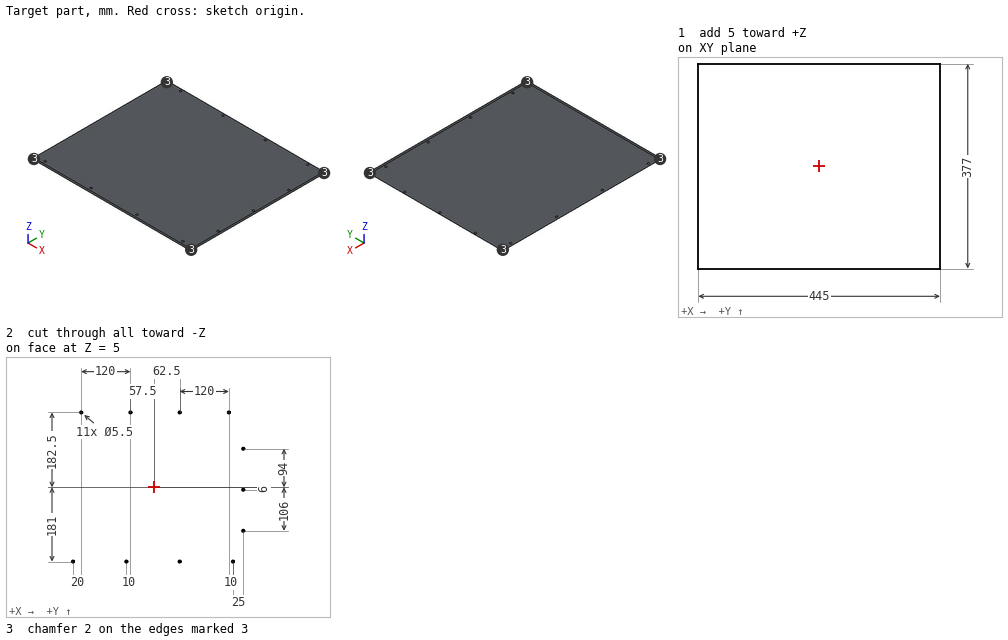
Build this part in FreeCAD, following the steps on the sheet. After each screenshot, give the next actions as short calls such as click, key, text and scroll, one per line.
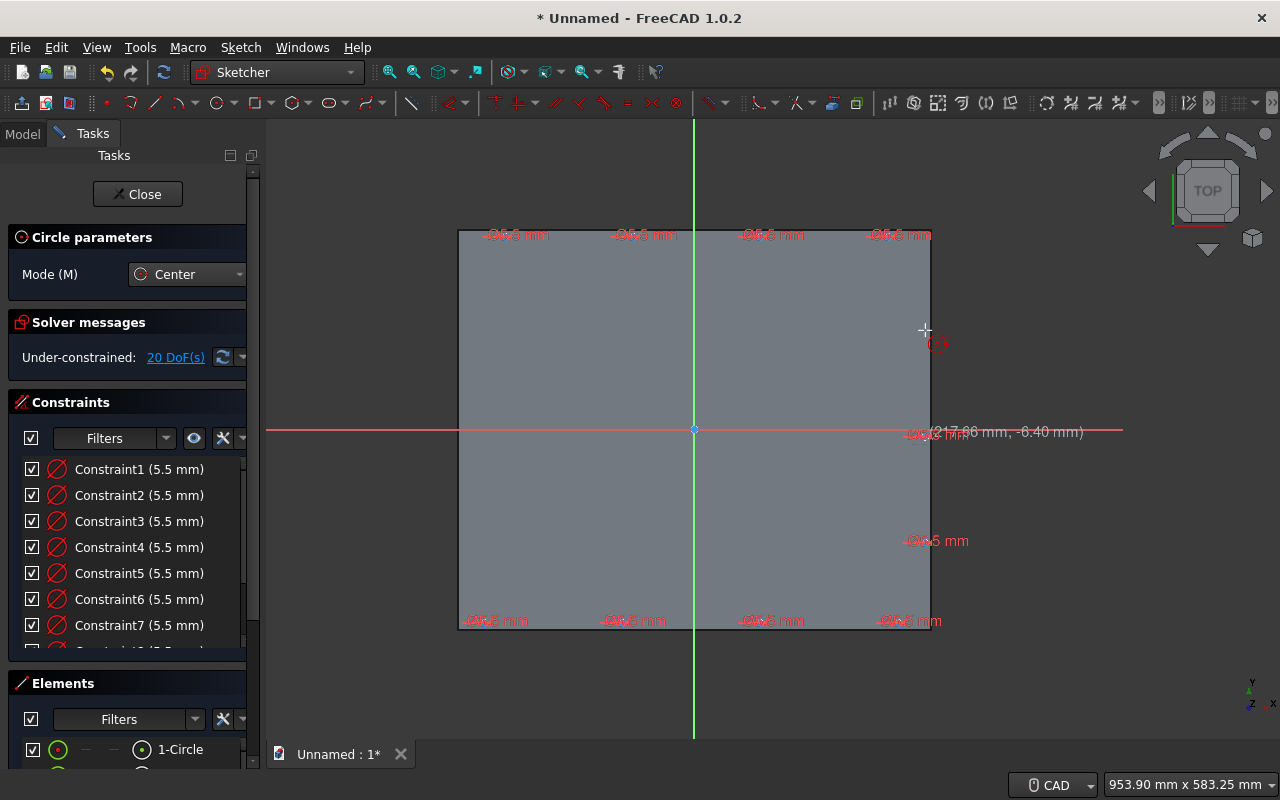
click(925, 330)
move(927, 328)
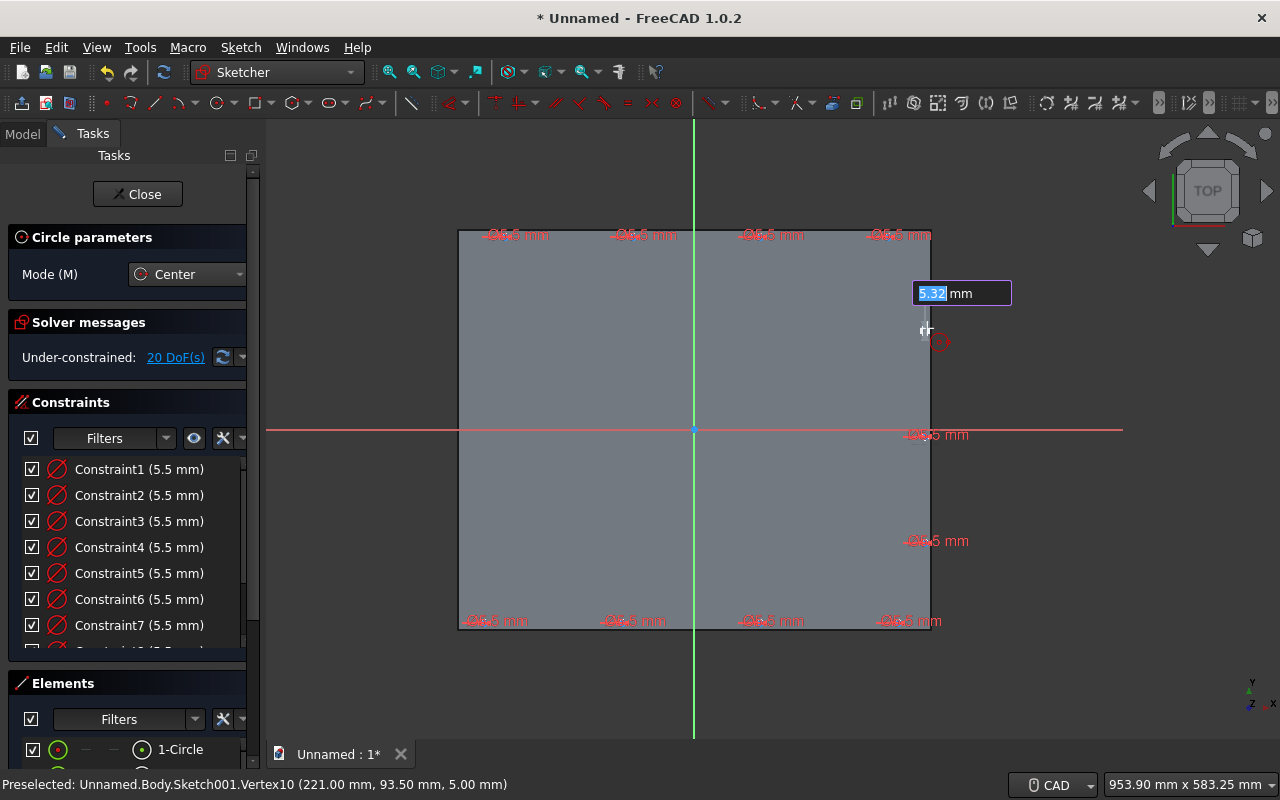
text(5.5)
key(Return)
key(Escape)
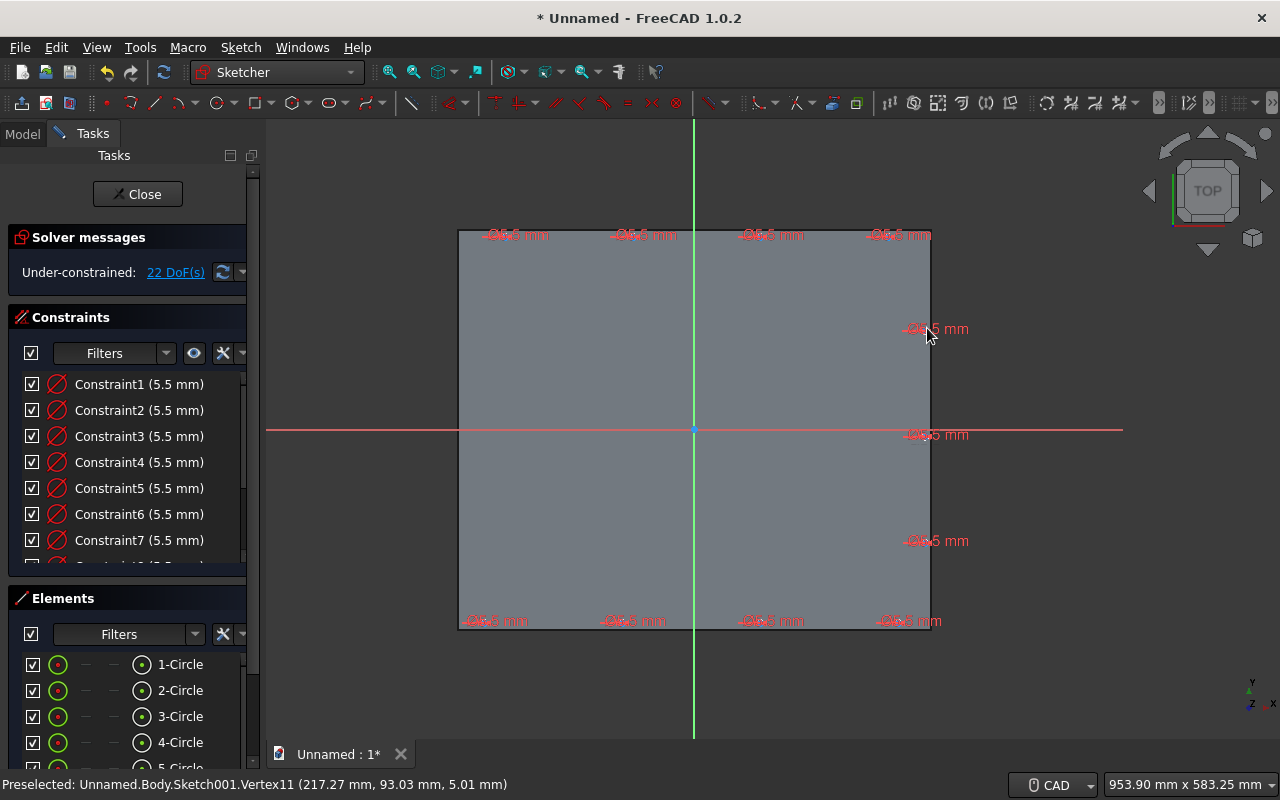
click(505, 237)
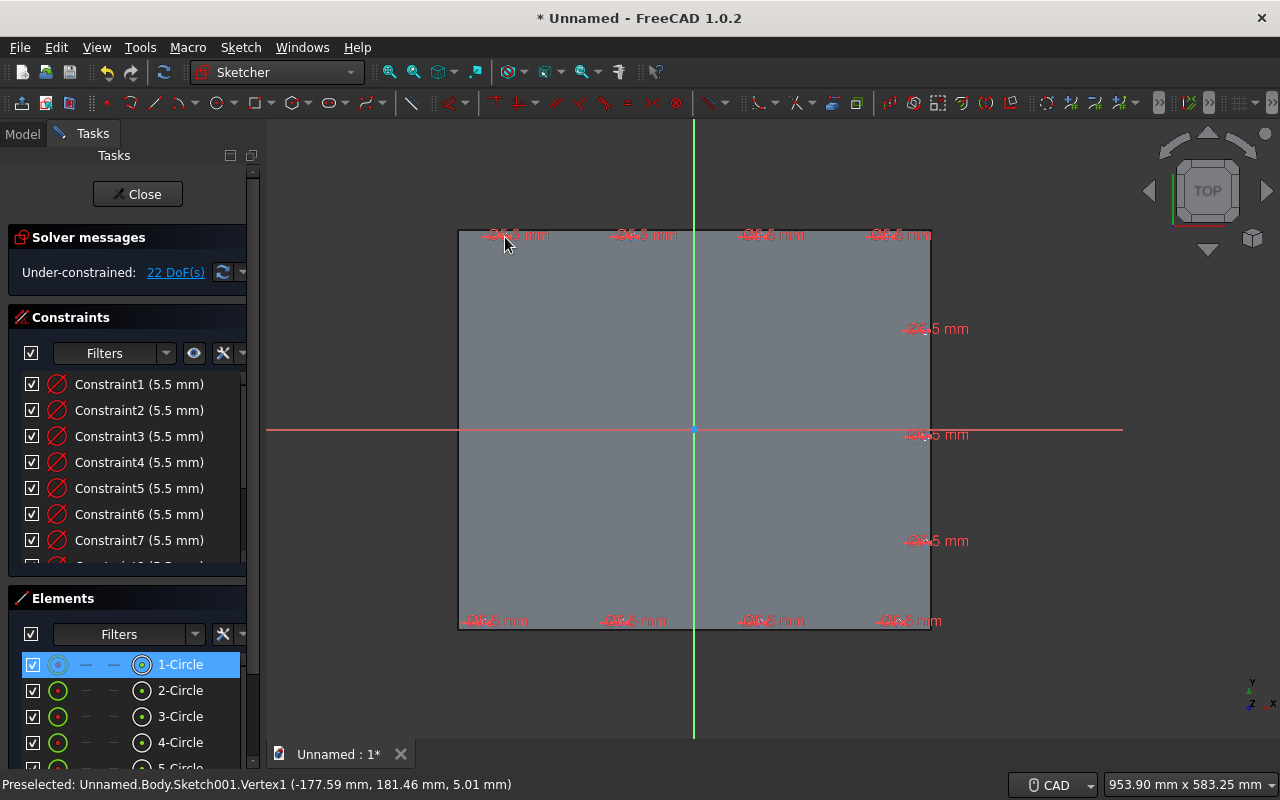
click(633, 237)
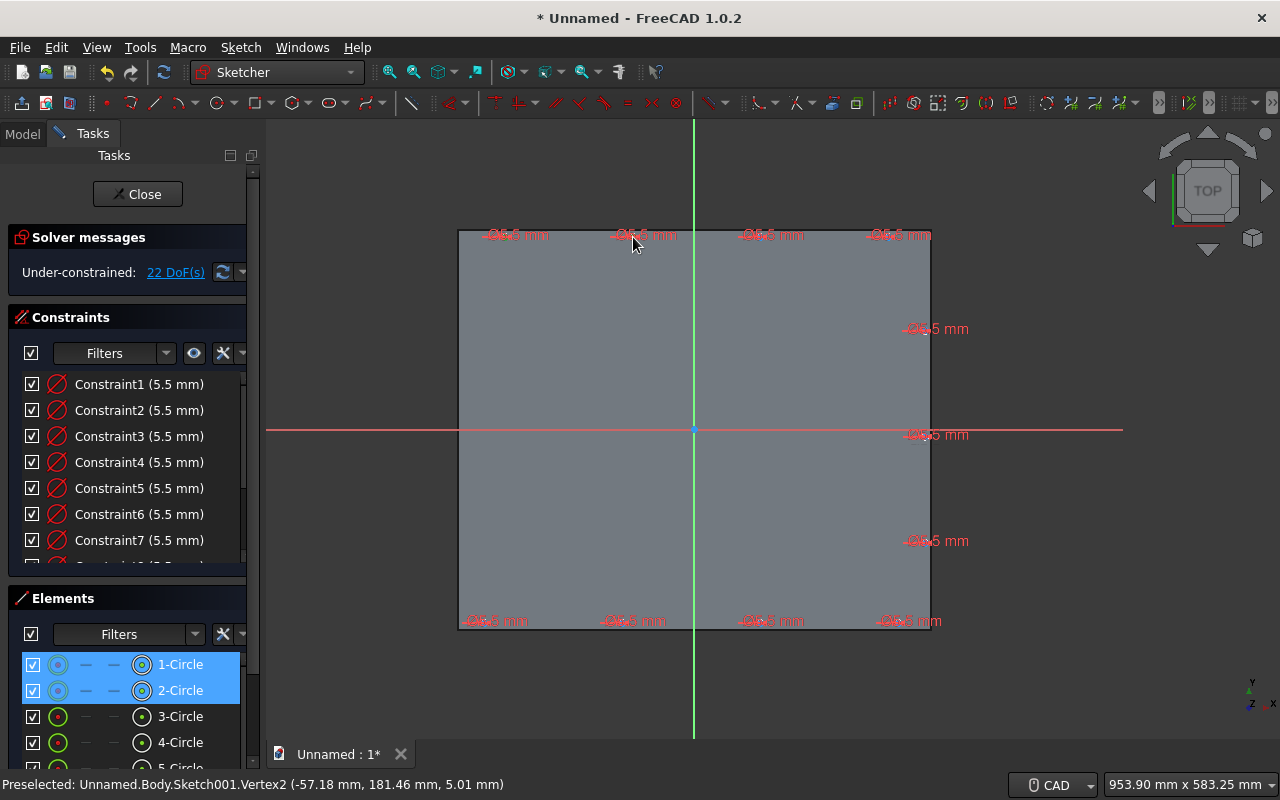
key(h)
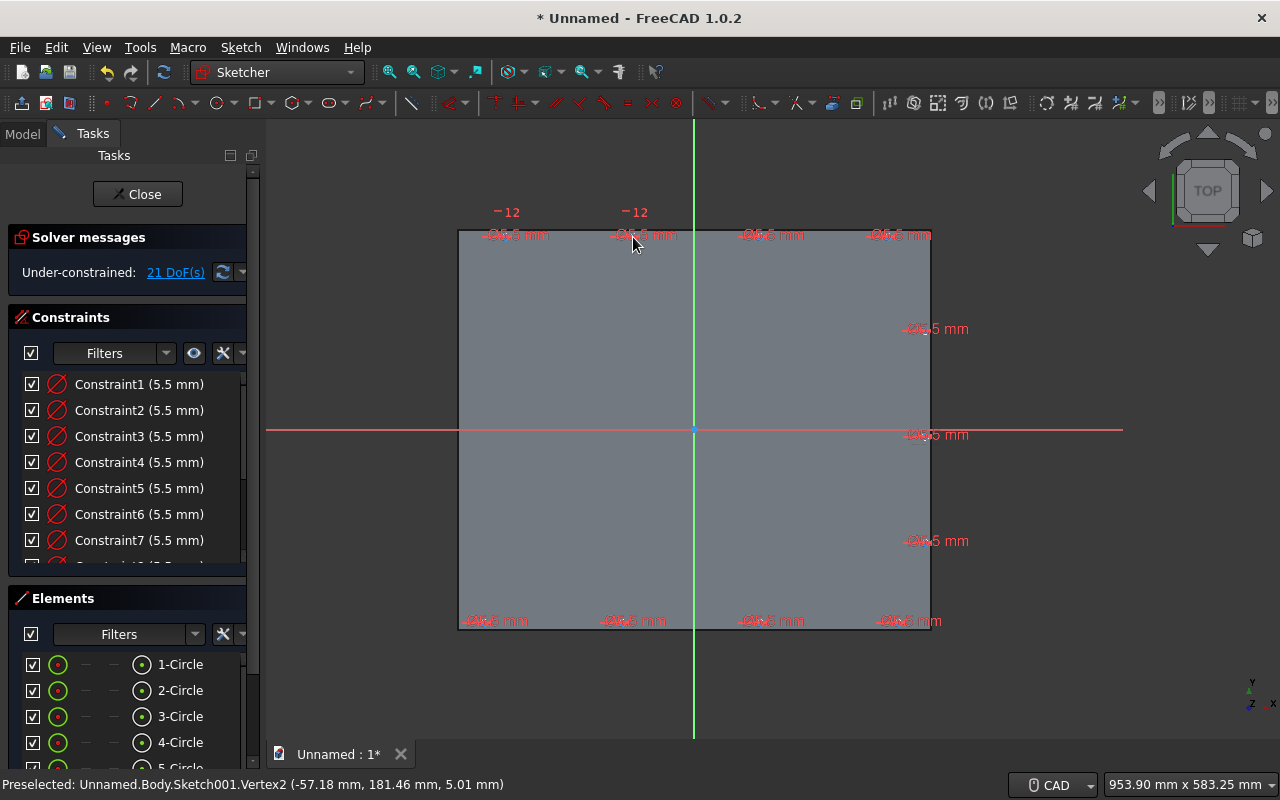
click(633, 237)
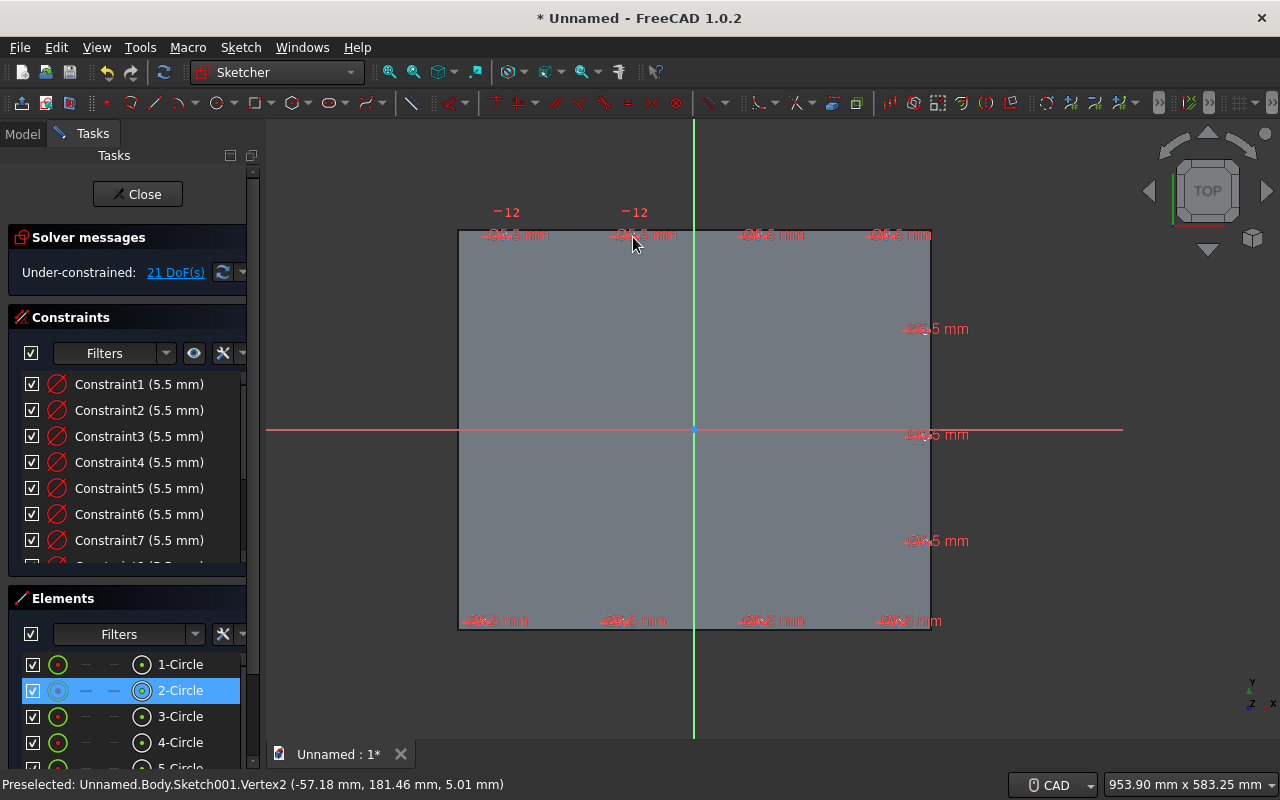
click(760, 237)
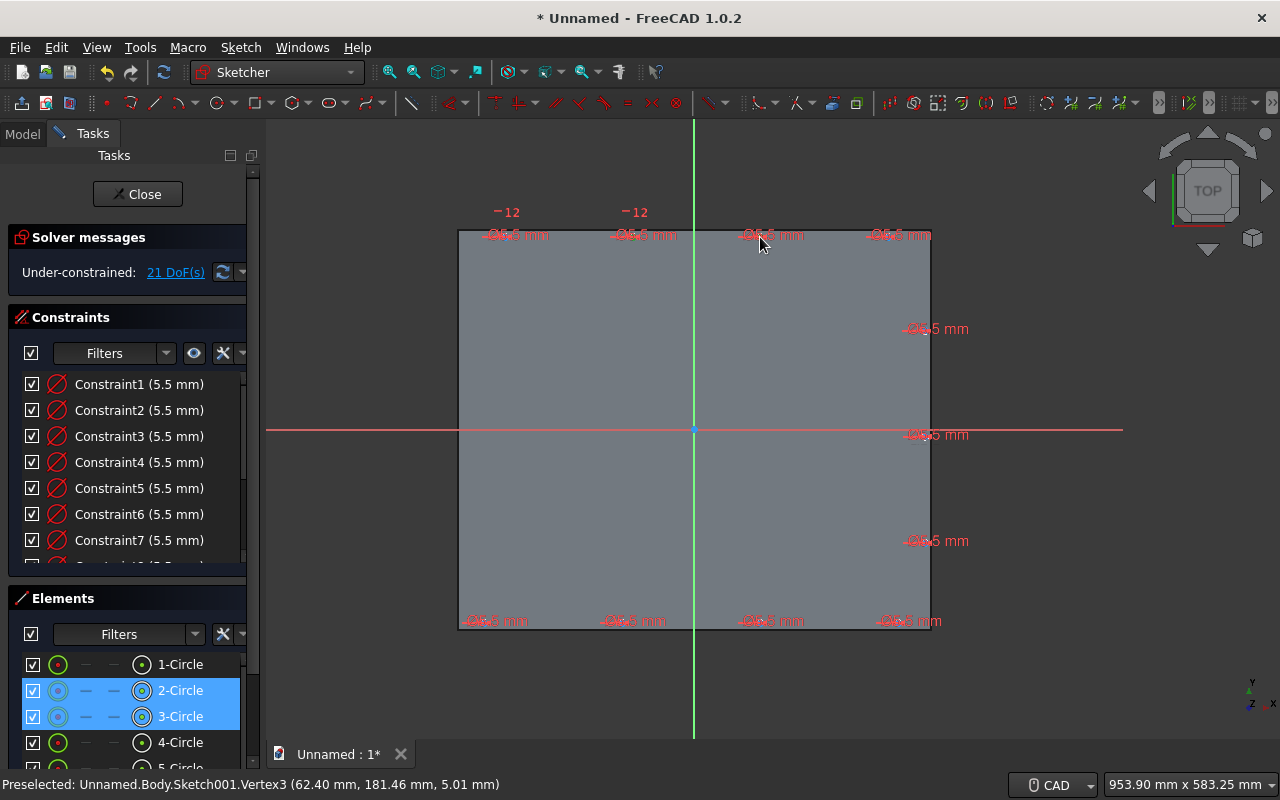
click(538, 104)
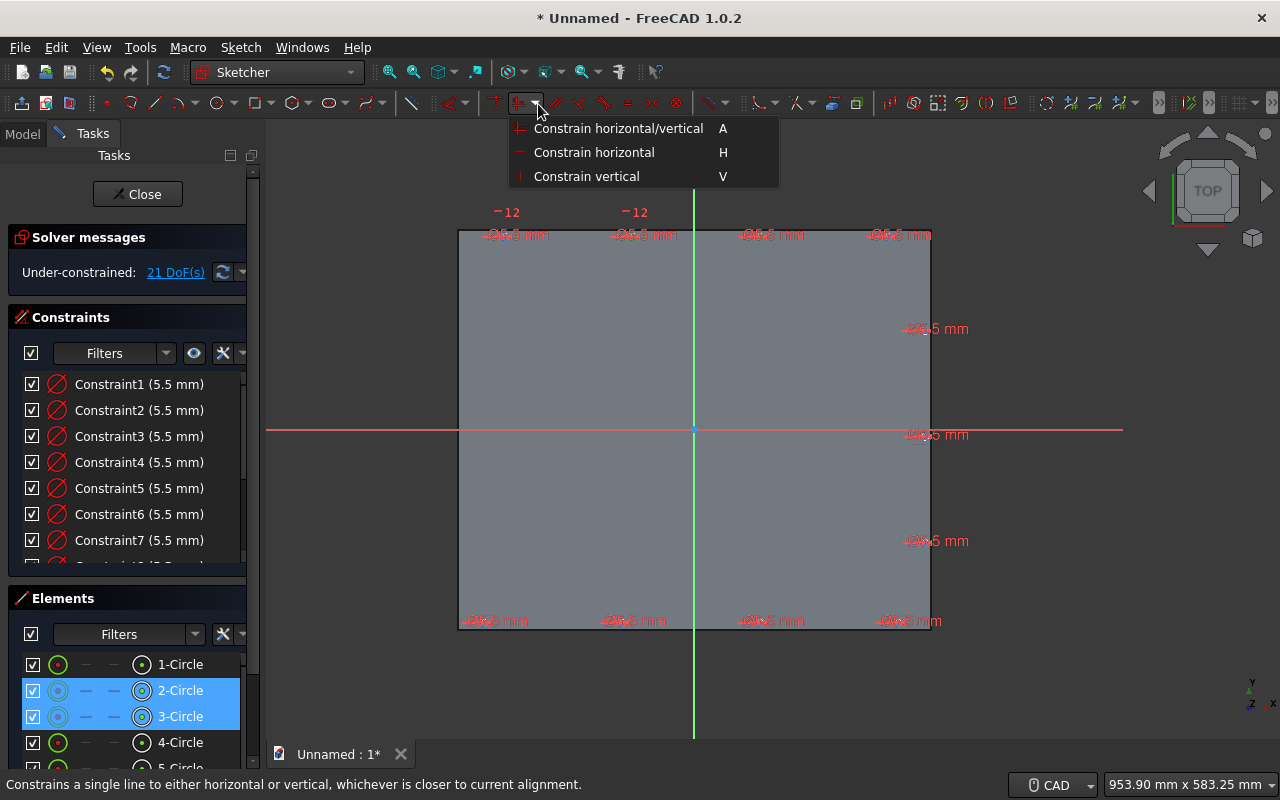
click(644, 152)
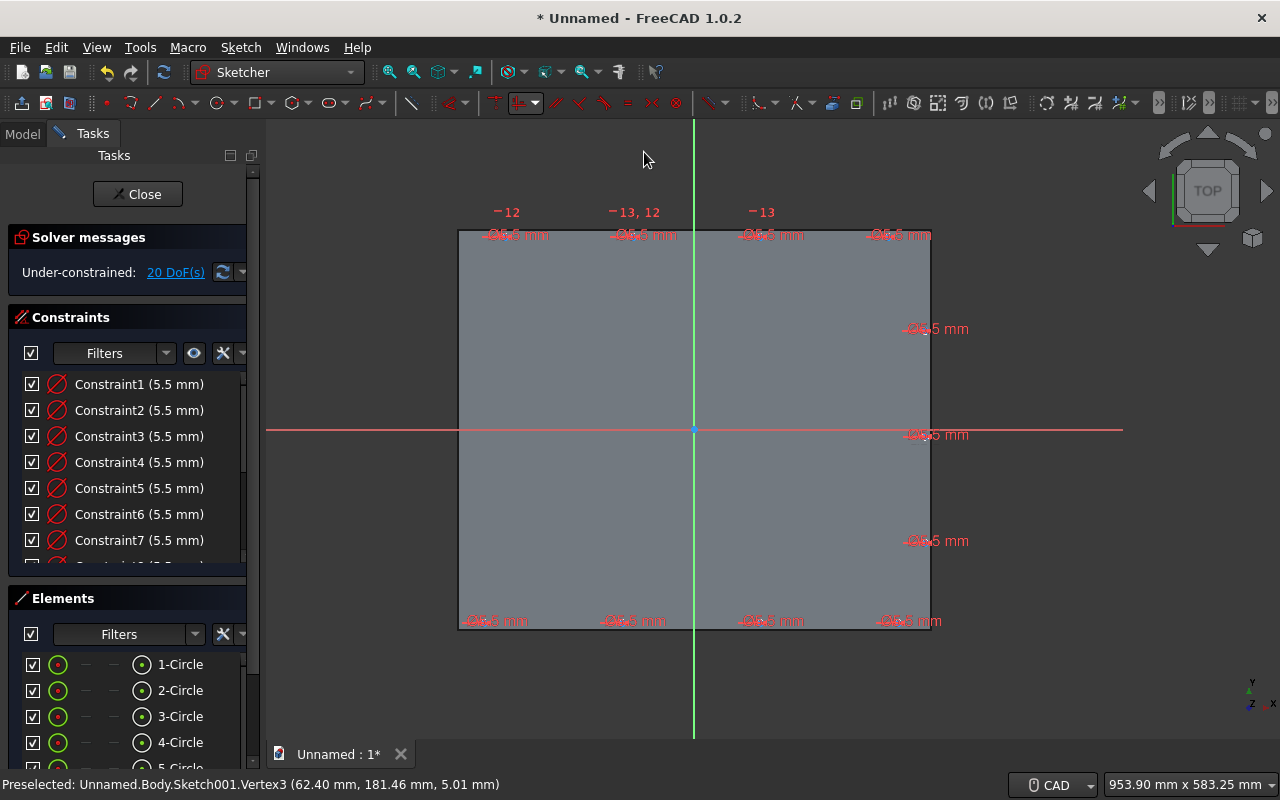
click(760, 237)